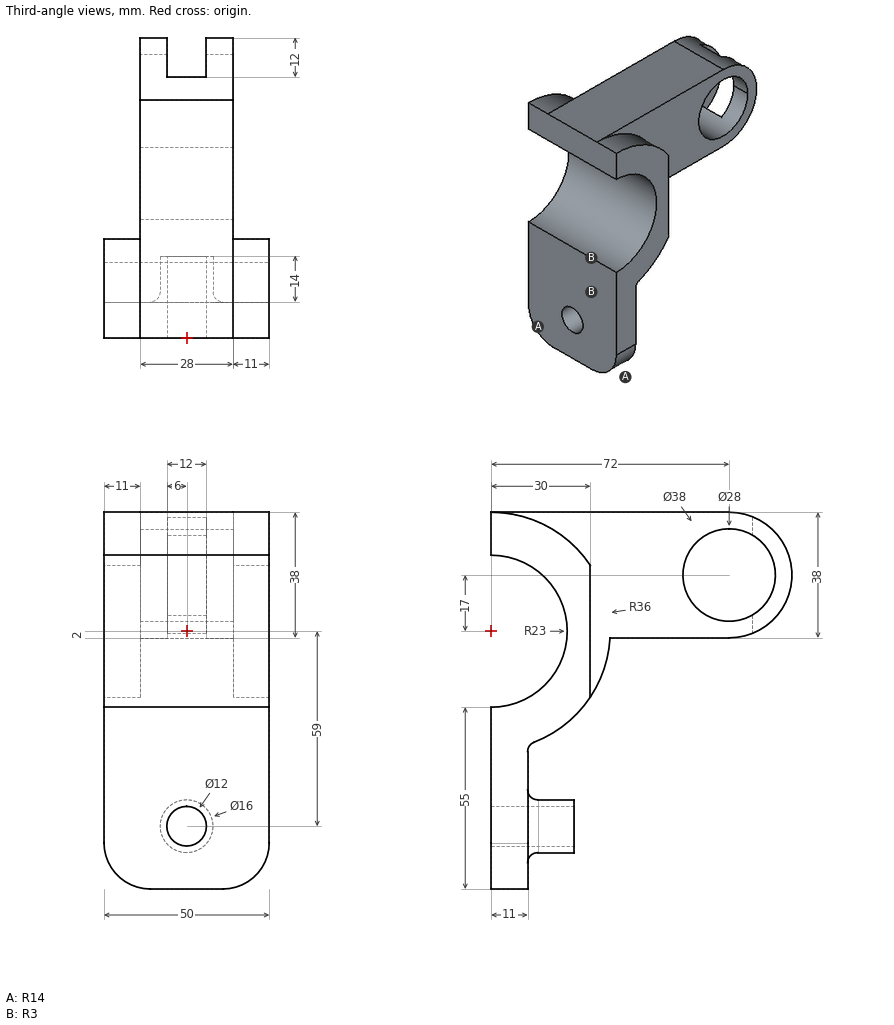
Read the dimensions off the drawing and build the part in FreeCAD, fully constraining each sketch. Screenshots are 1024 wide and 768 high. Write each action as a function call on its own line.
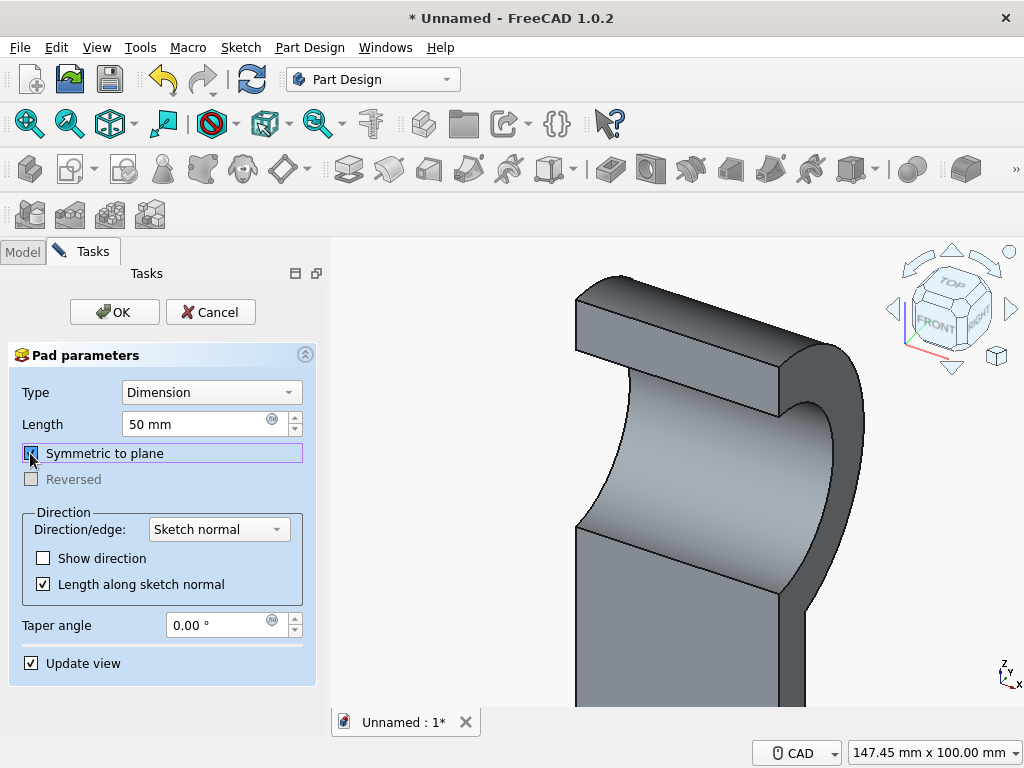
click(115, 312)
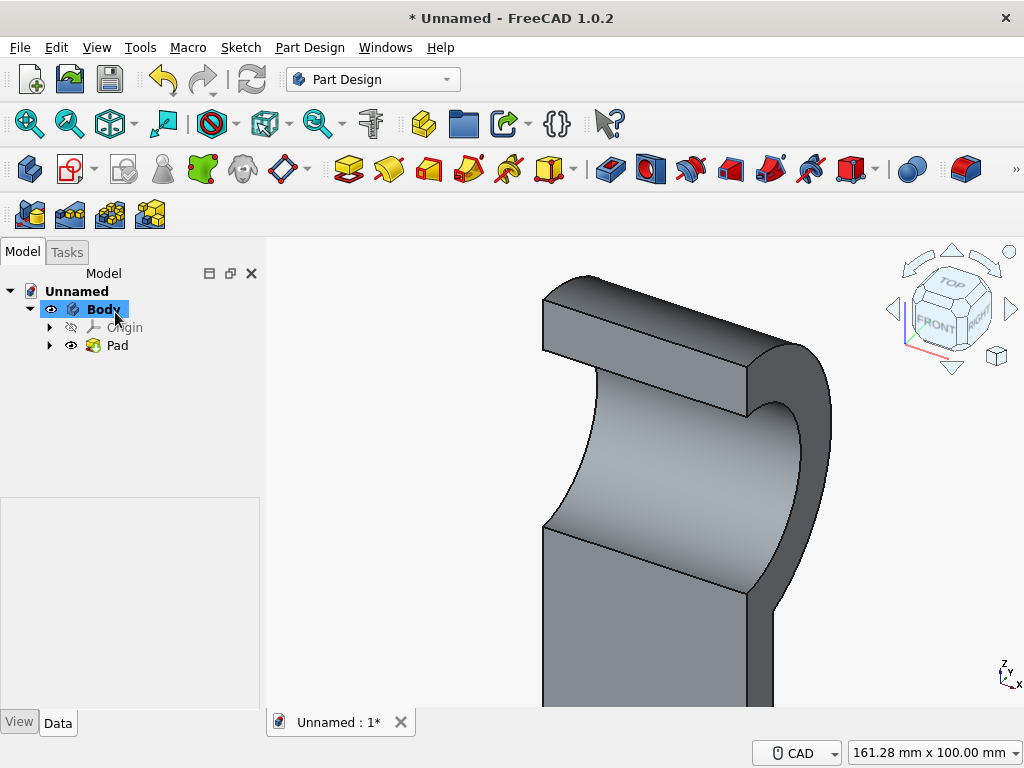
click(30, 124)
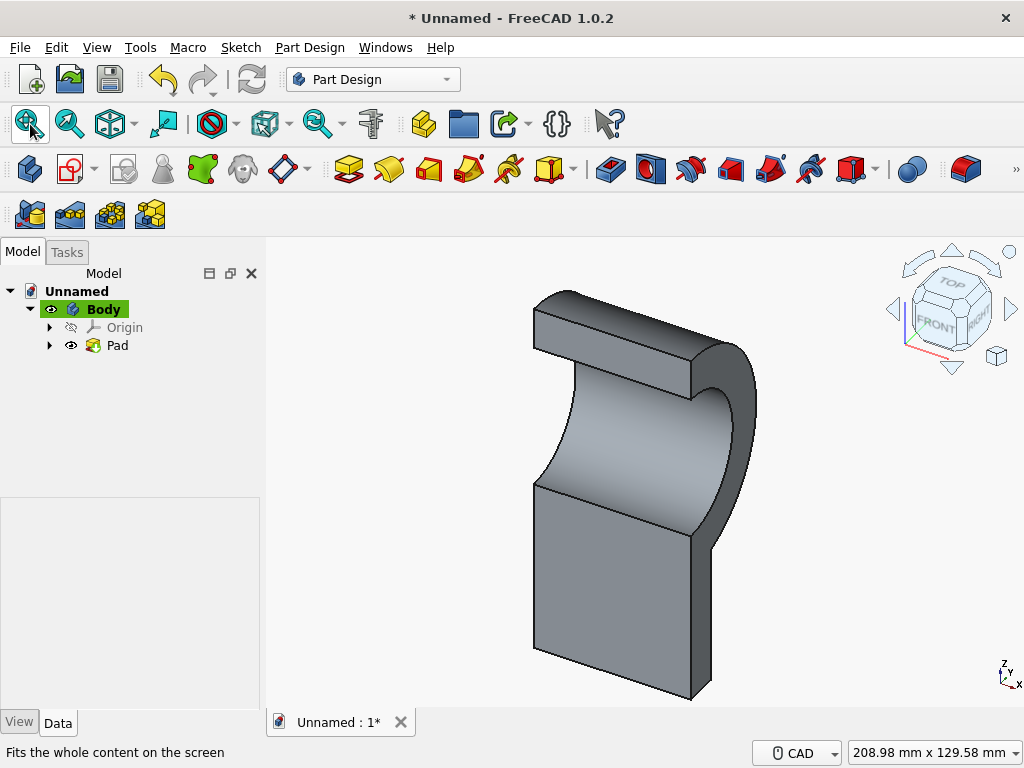
key(0)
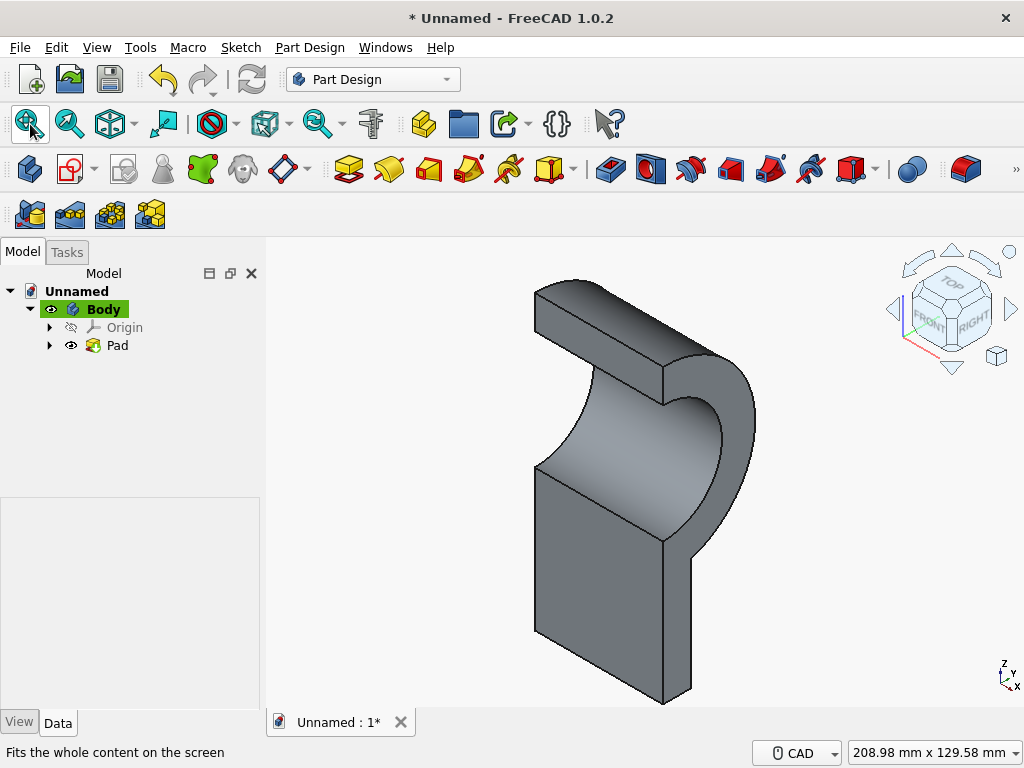
key(2)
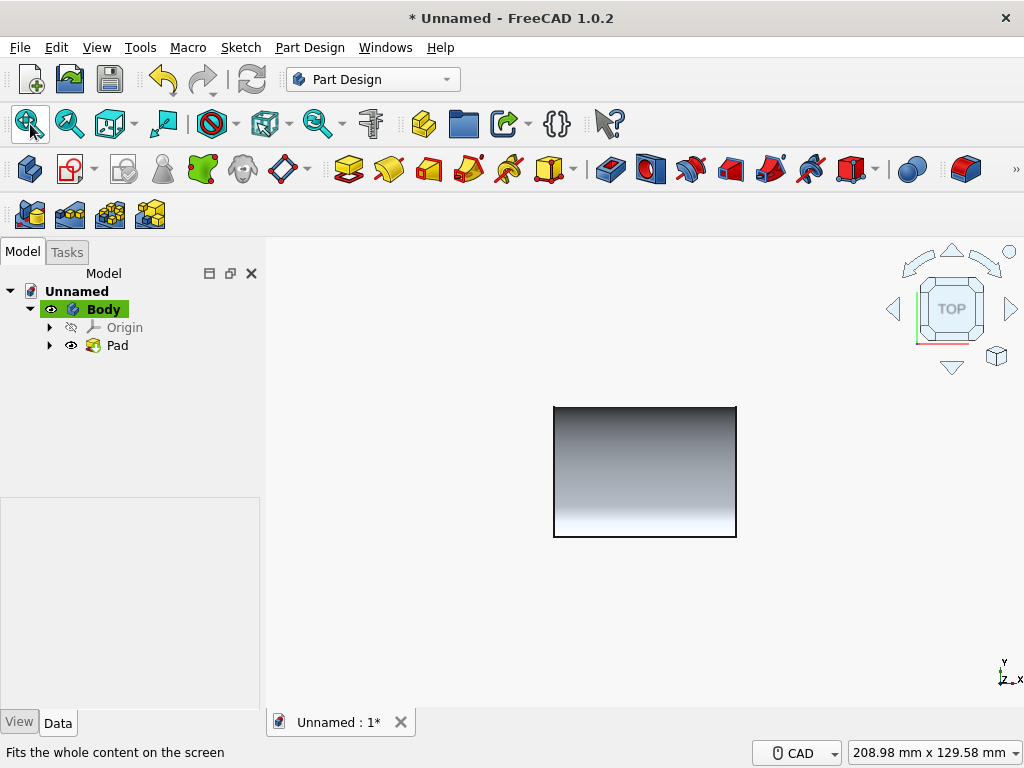
click(30, 124)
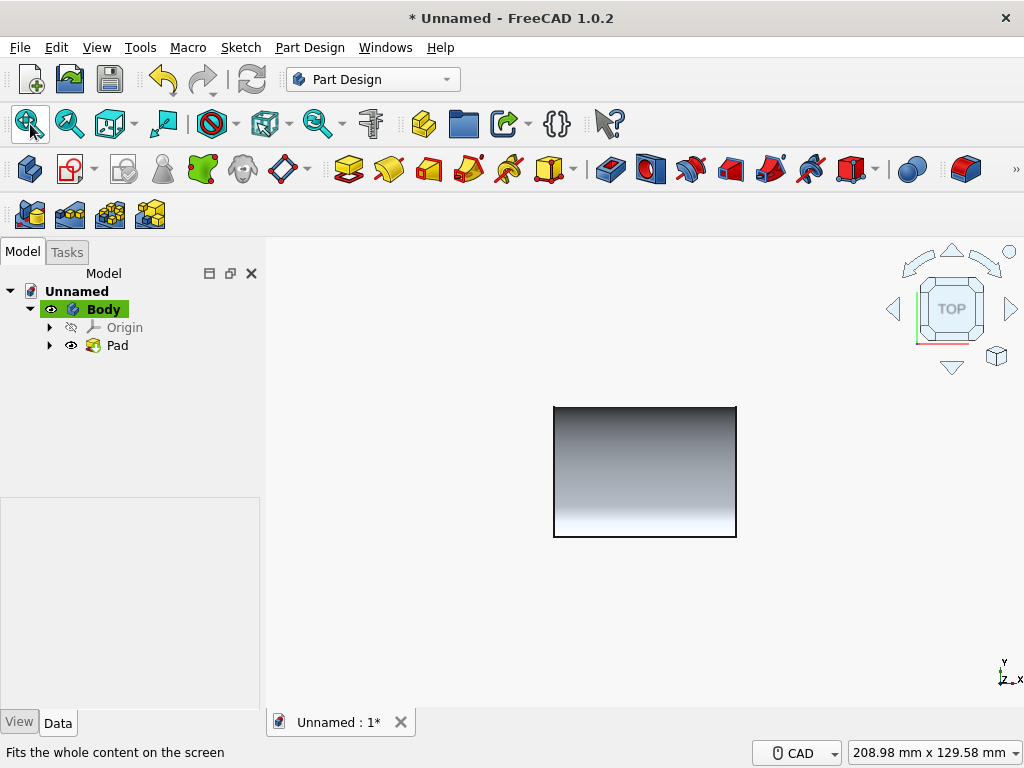
key(1)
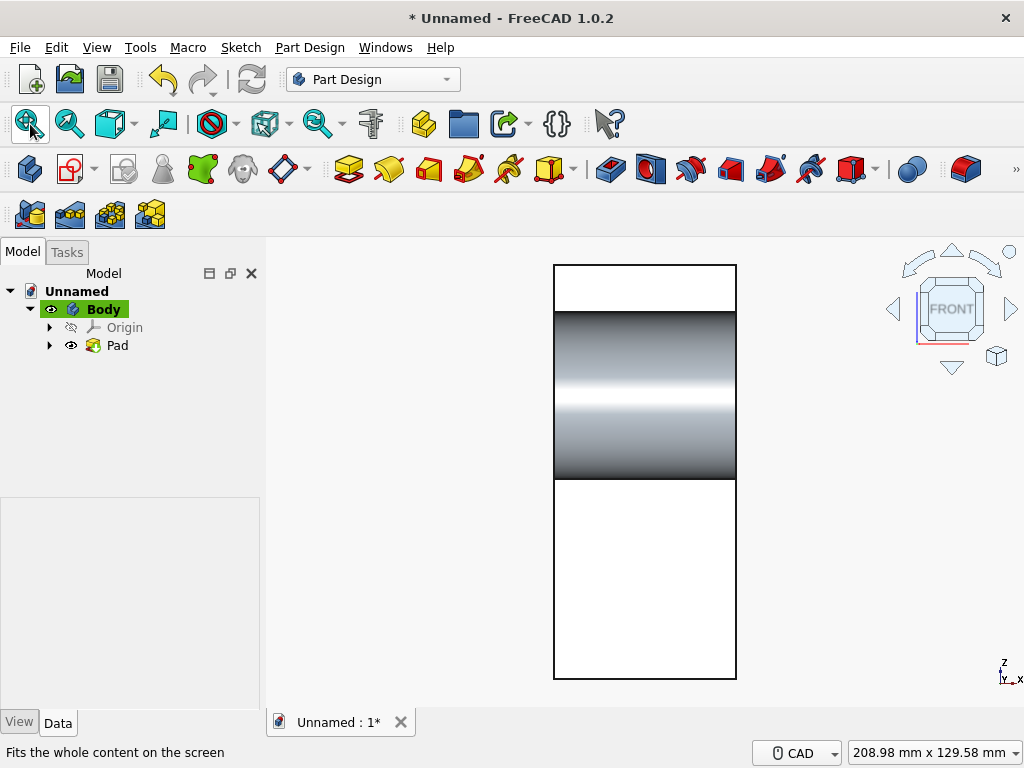
key(3)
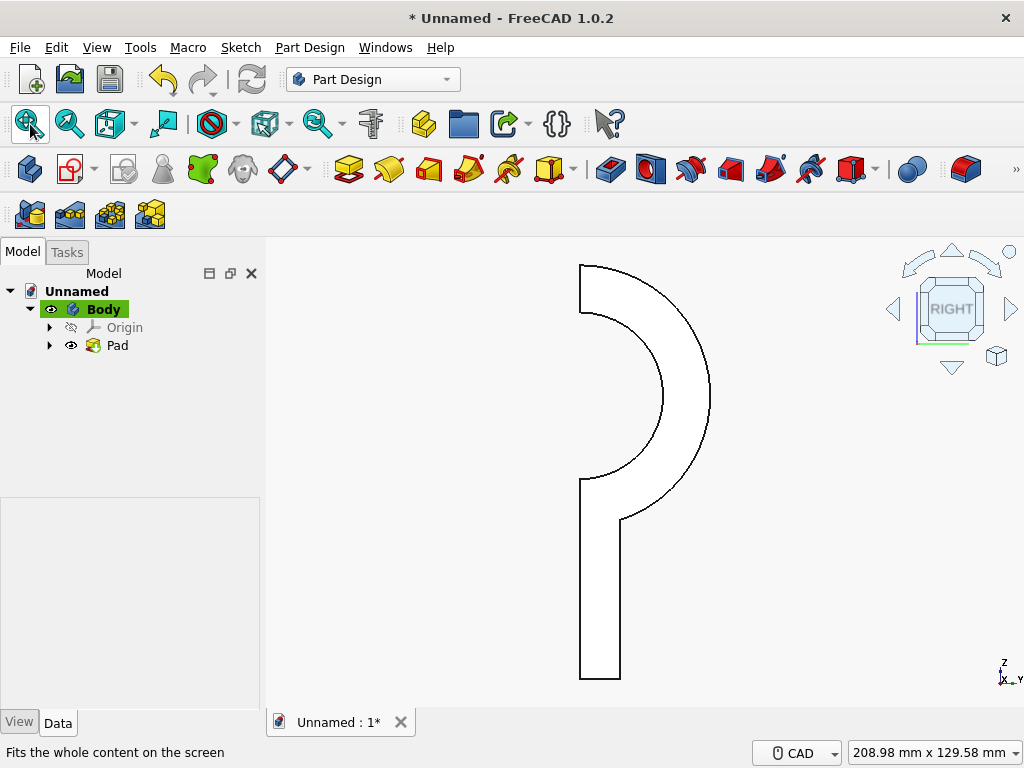
click(600, 678)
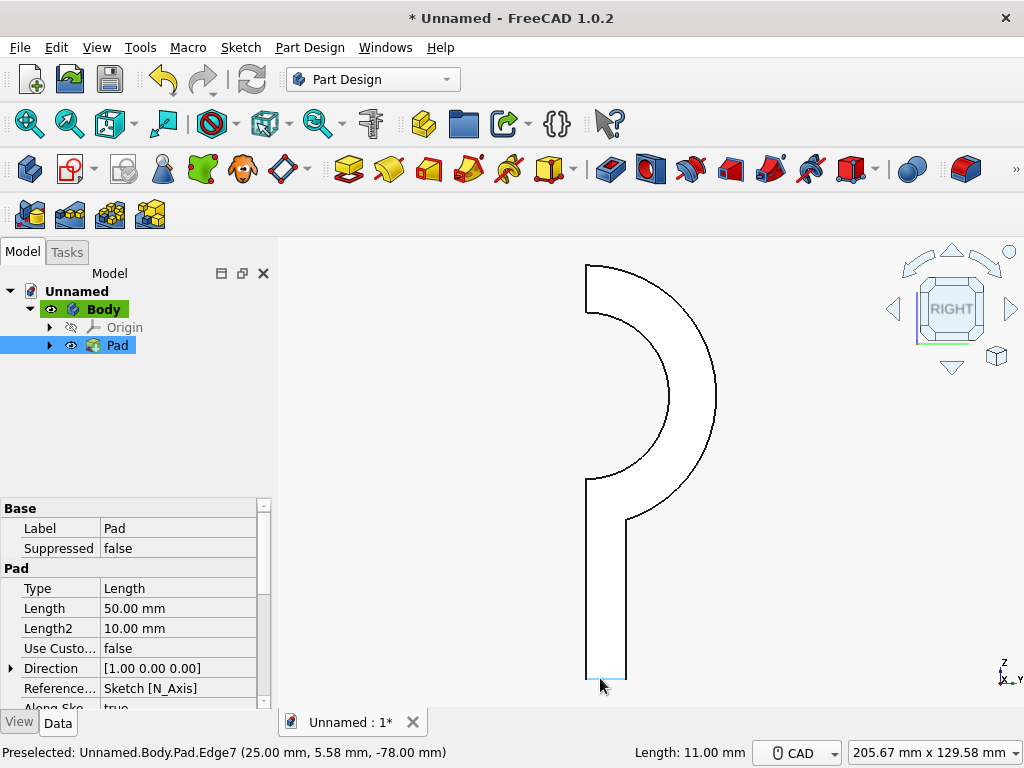
key(5)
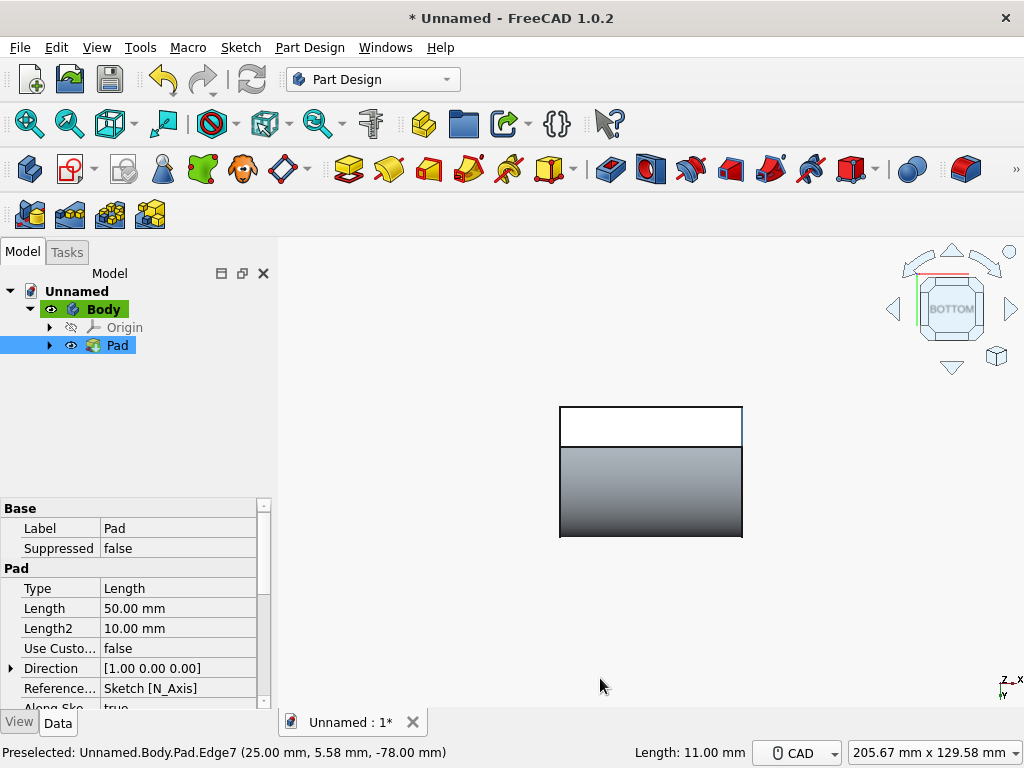
click(30, 124)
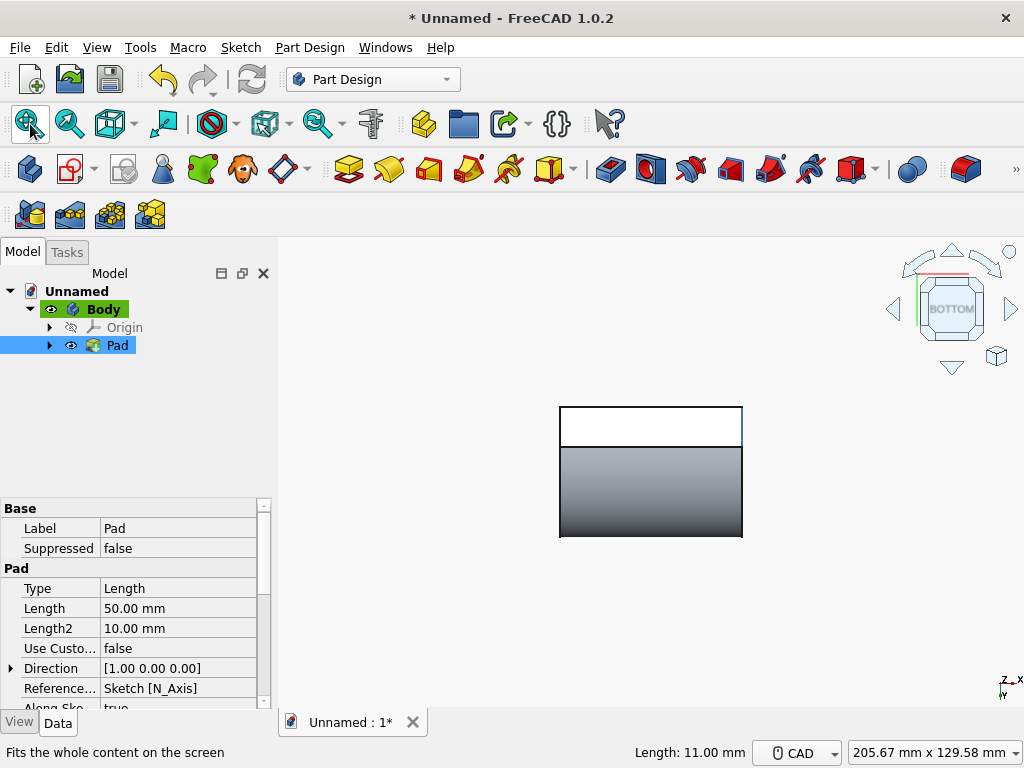
click(560, 426, ctrl)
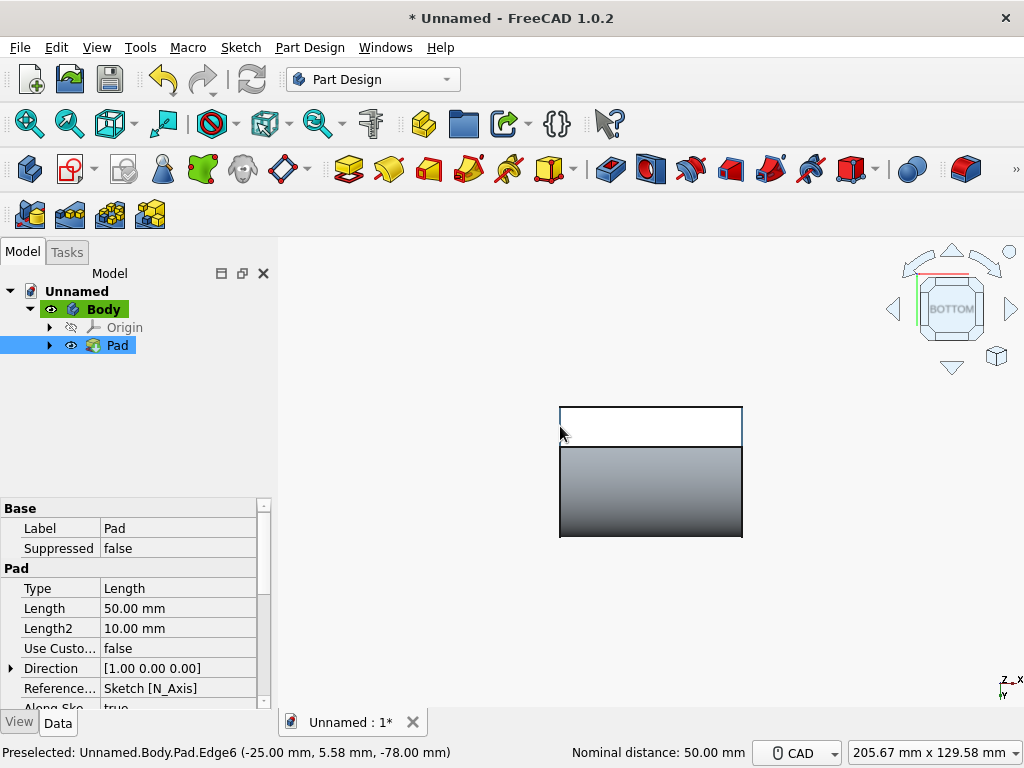
click(966, 170)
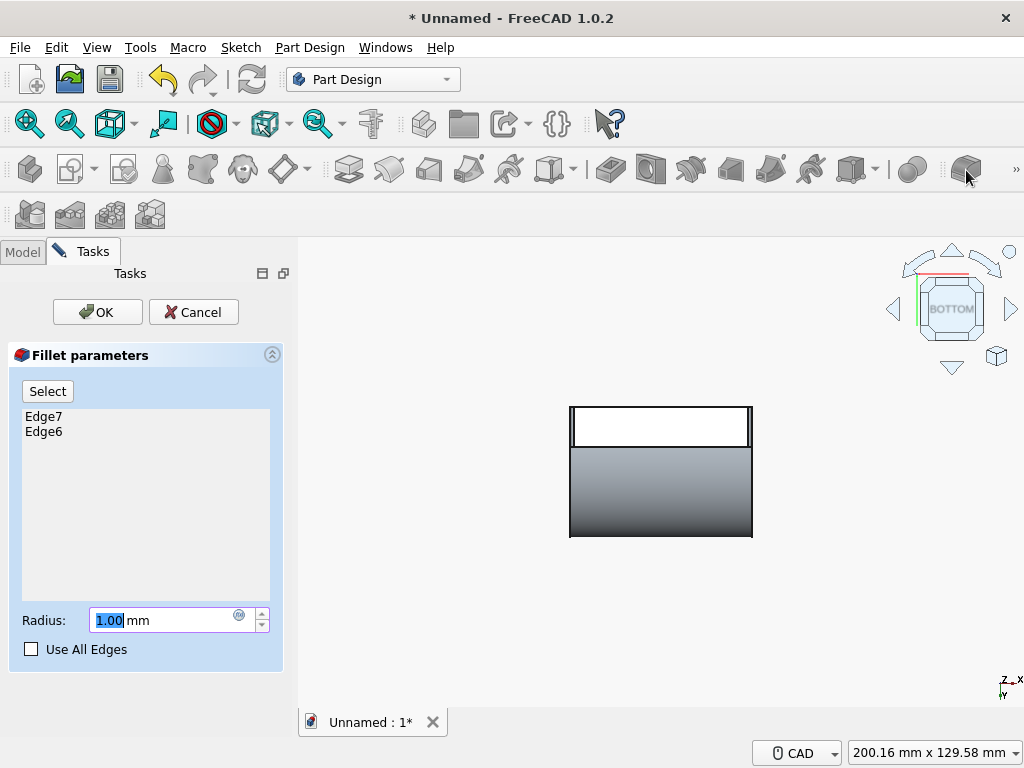
text(14)
key(Tab)